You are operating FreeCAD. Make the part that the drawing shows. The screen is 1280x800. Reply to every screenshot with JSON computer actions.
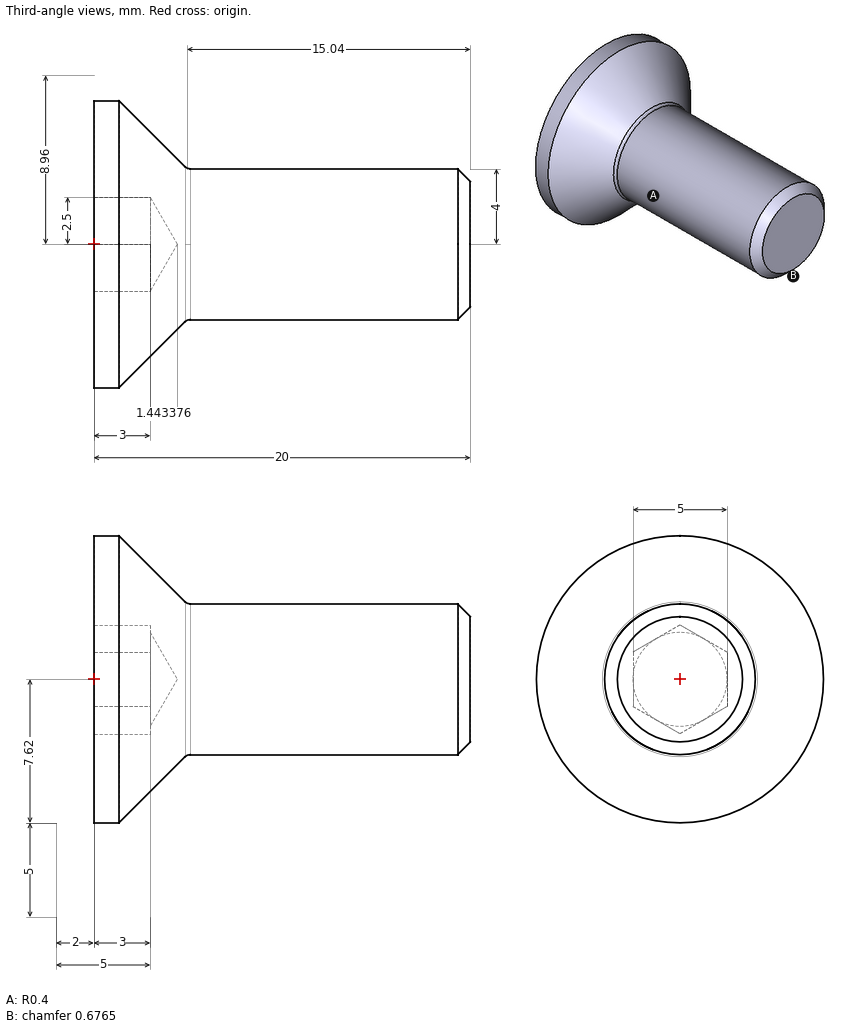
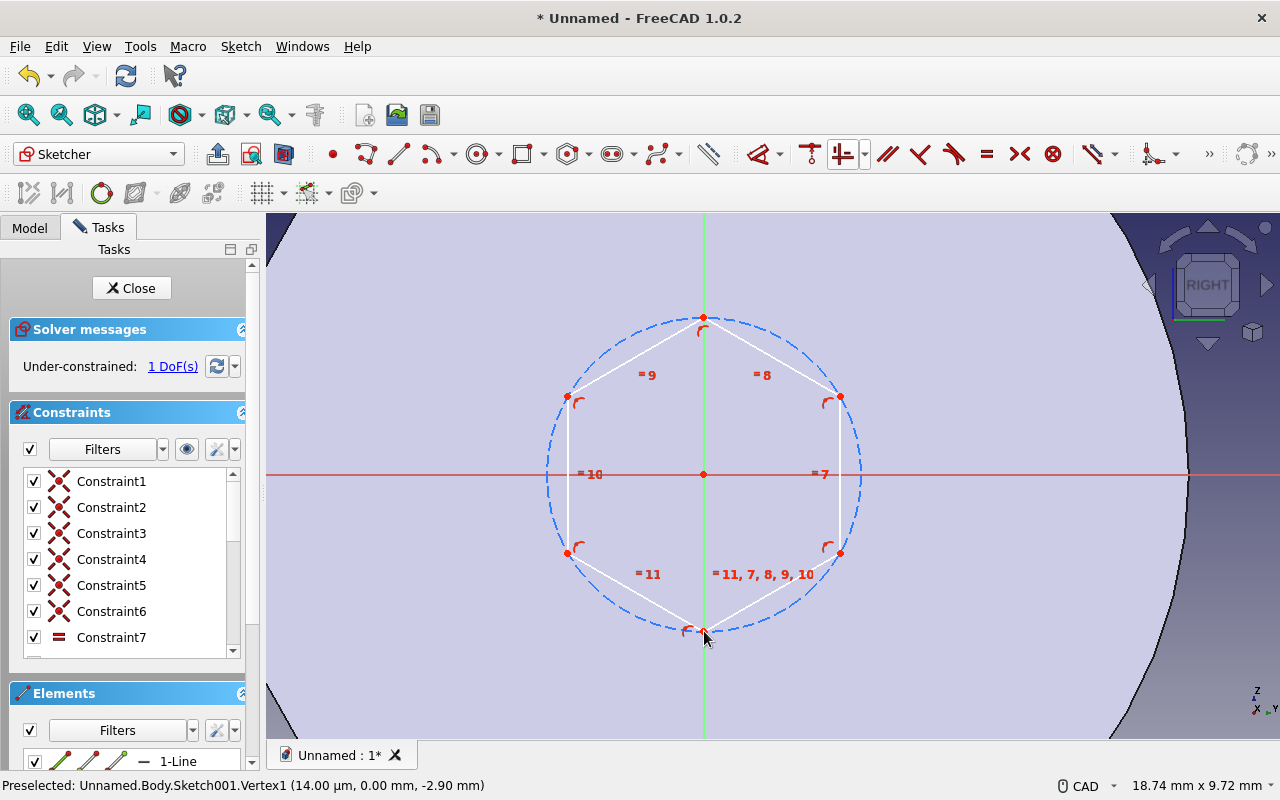
{"action": "left_click", "coordinate": [758, 154]}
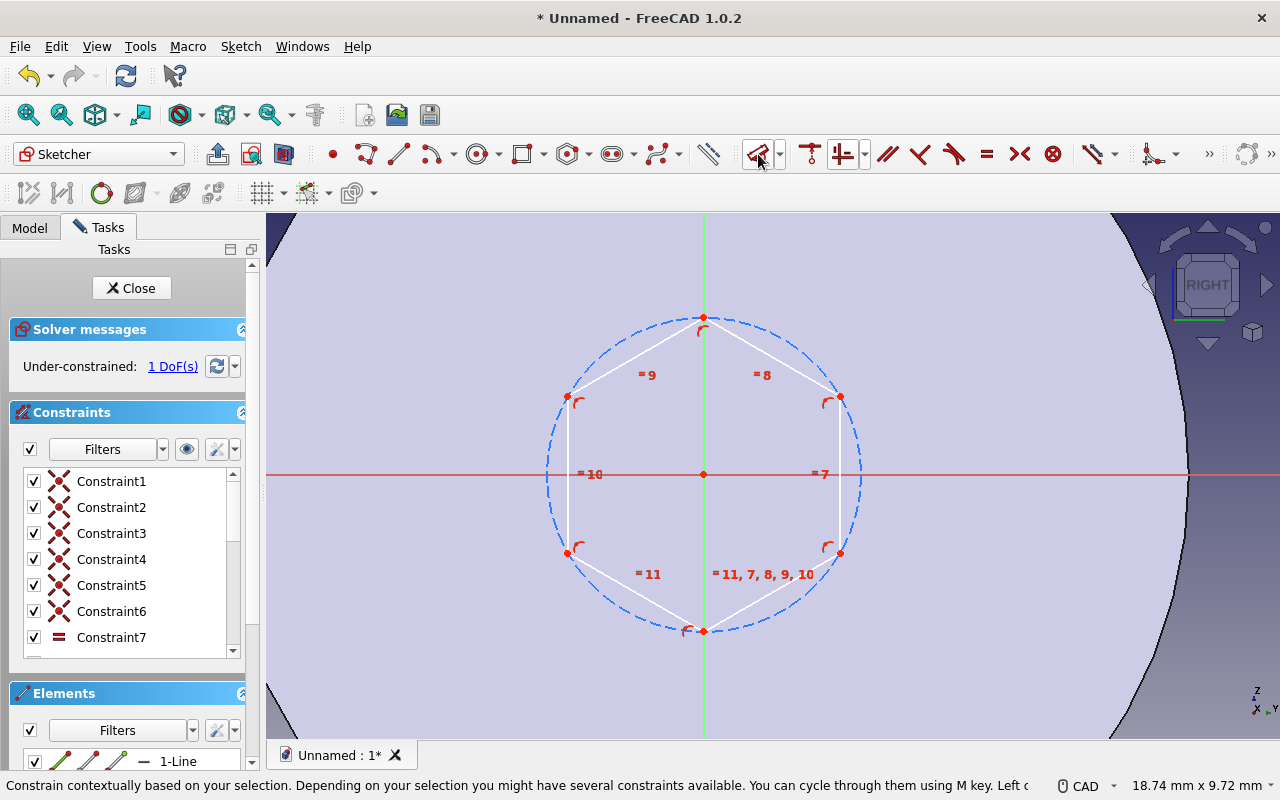
{"action": "left_click", "coordinate": [568, 396]}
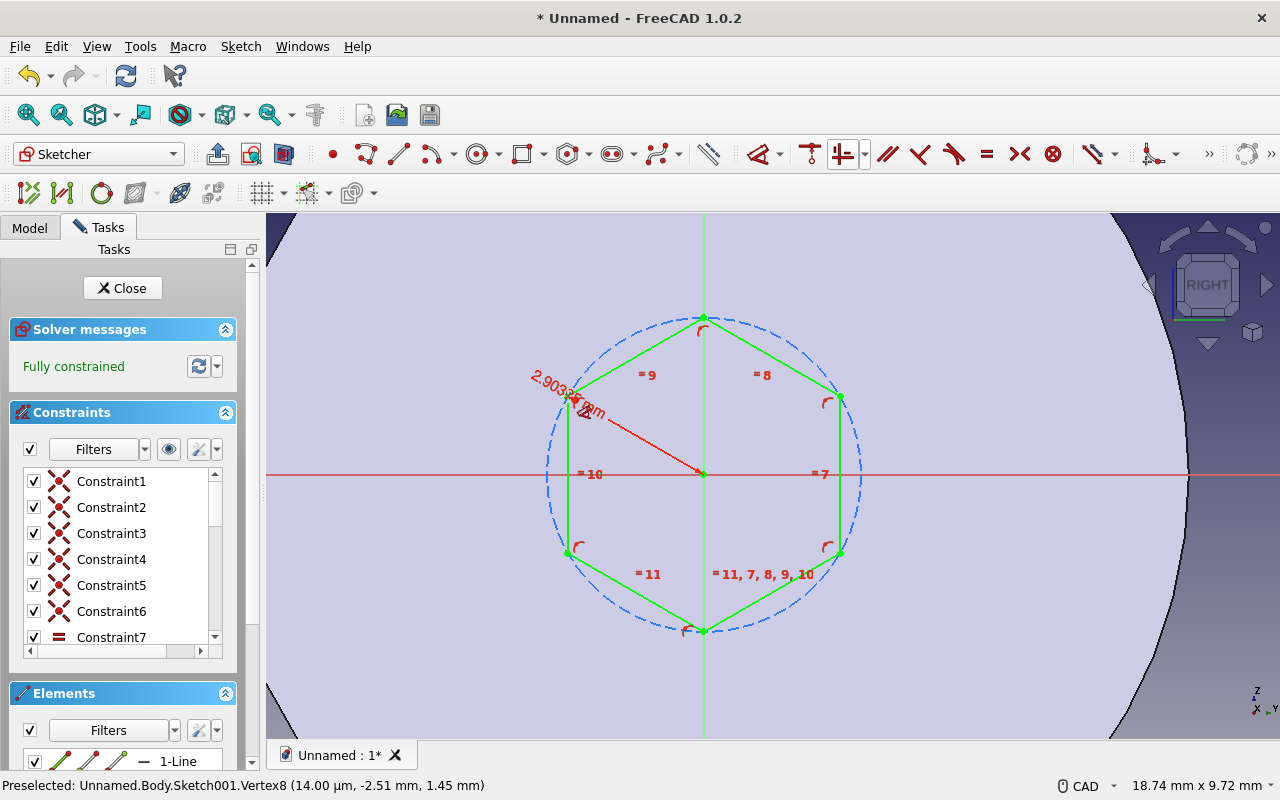
{"action": "left_click", "coordinate": [840, 553]}
{"action": "left_click", "coordinate": [641, 314]}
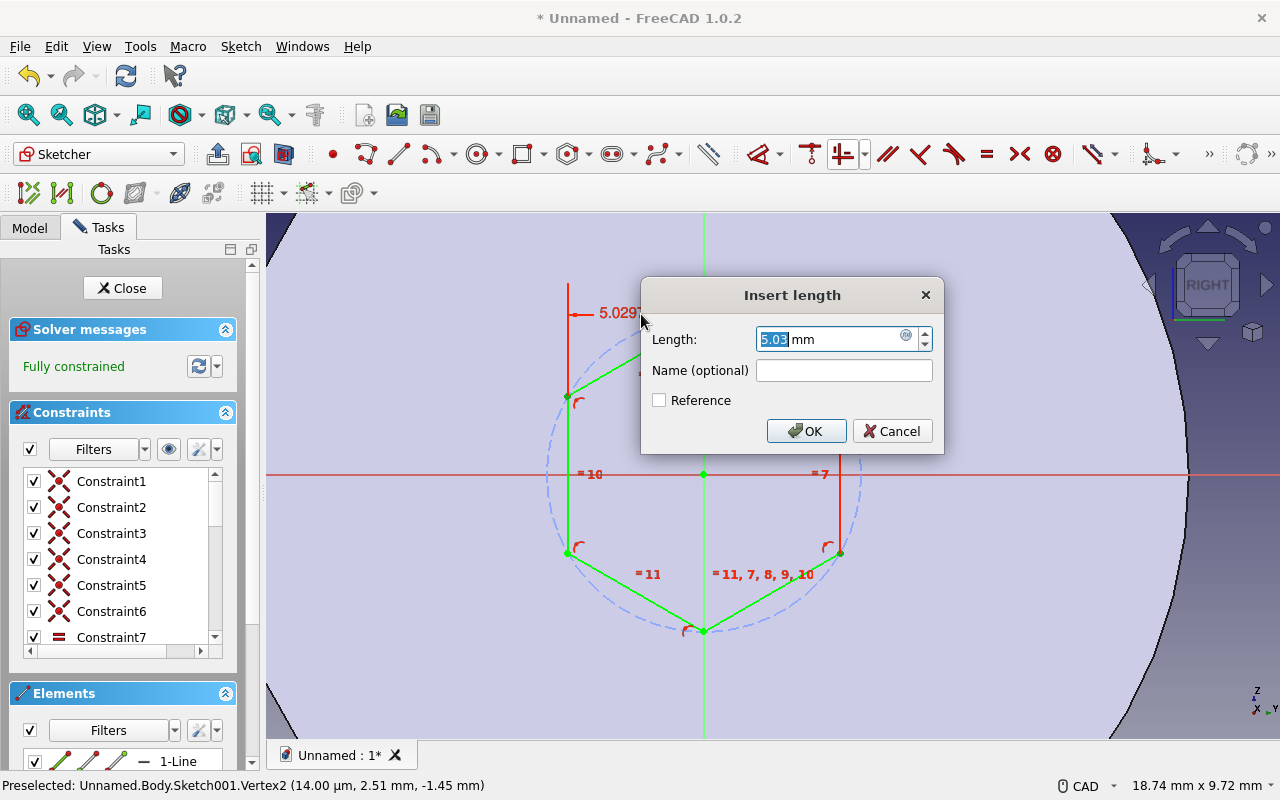
{"action": "type", "text": "5"}
{"action": "key", "text": "Return"}
{"action": "key", "text": "Escape"}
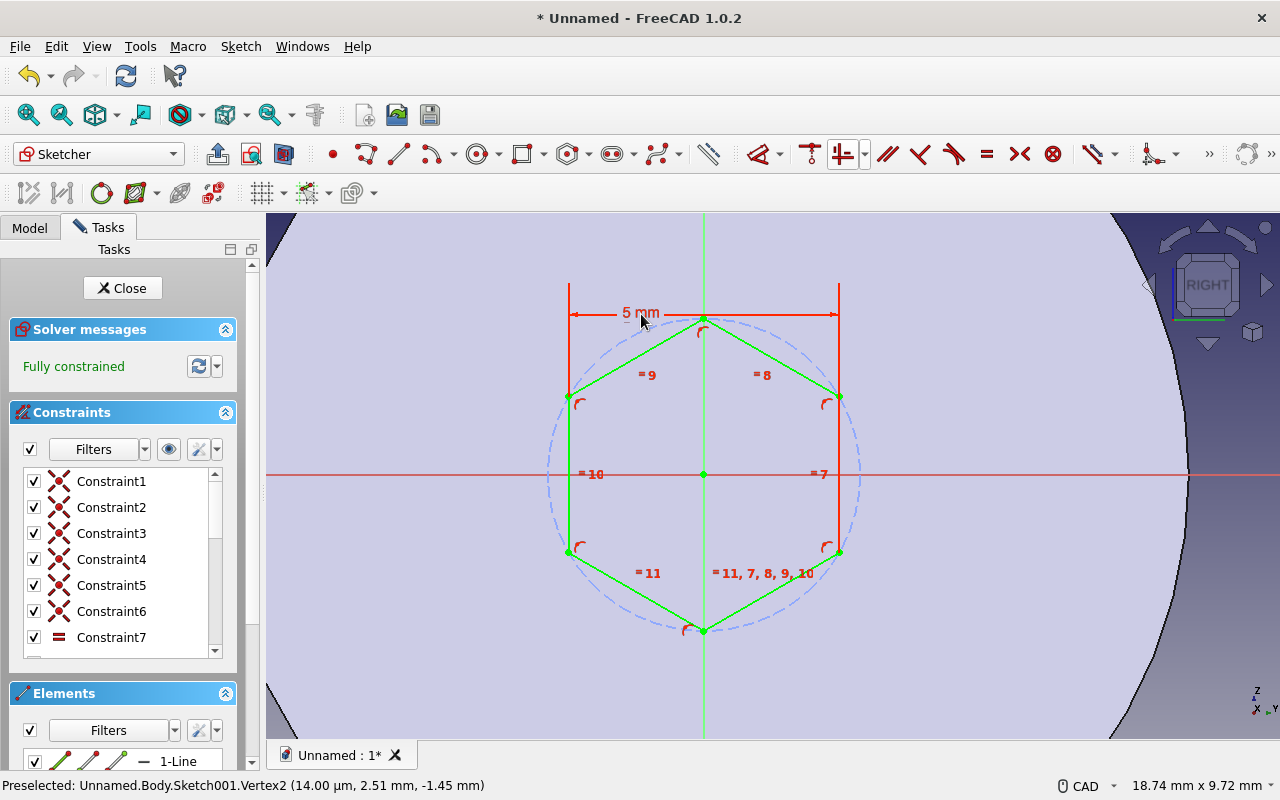
{"action": "left_click", "coordinate": [123, 288]}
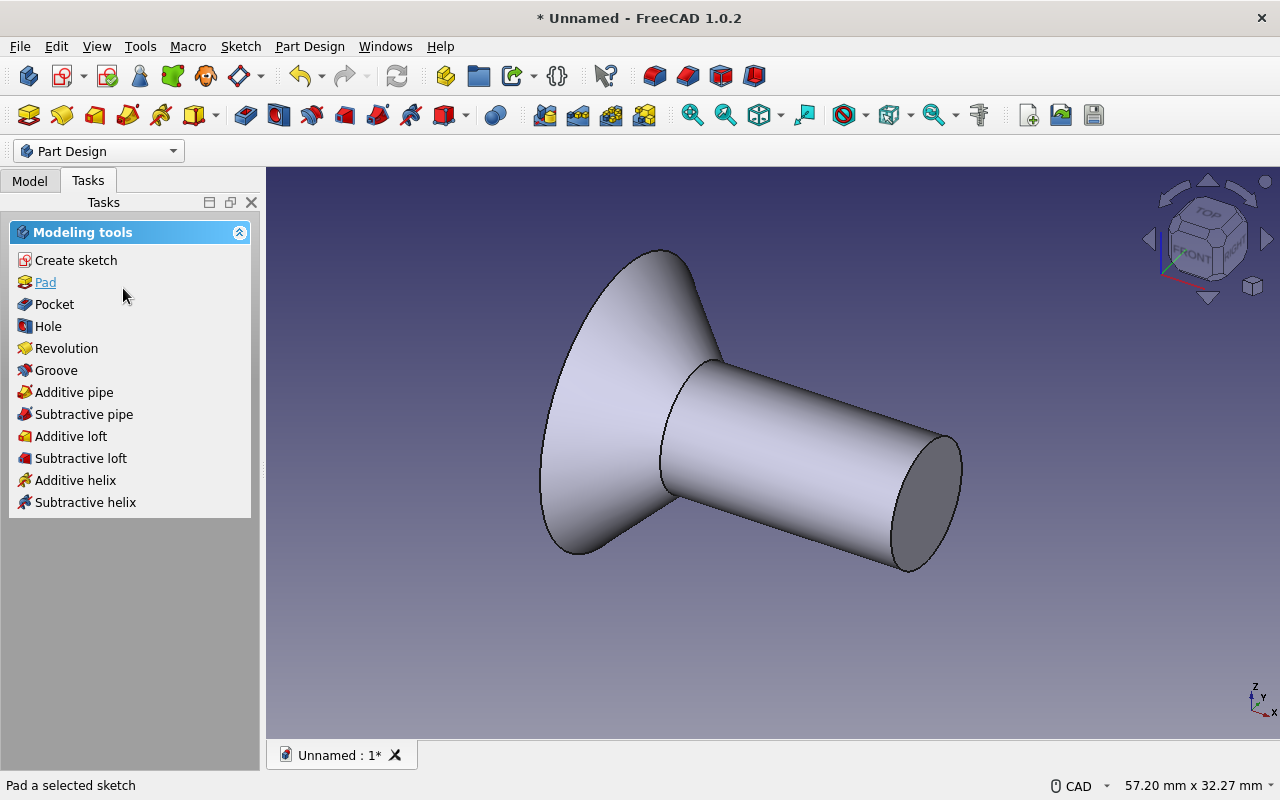
{"action": "left_click", "coordinate": [246, 116]}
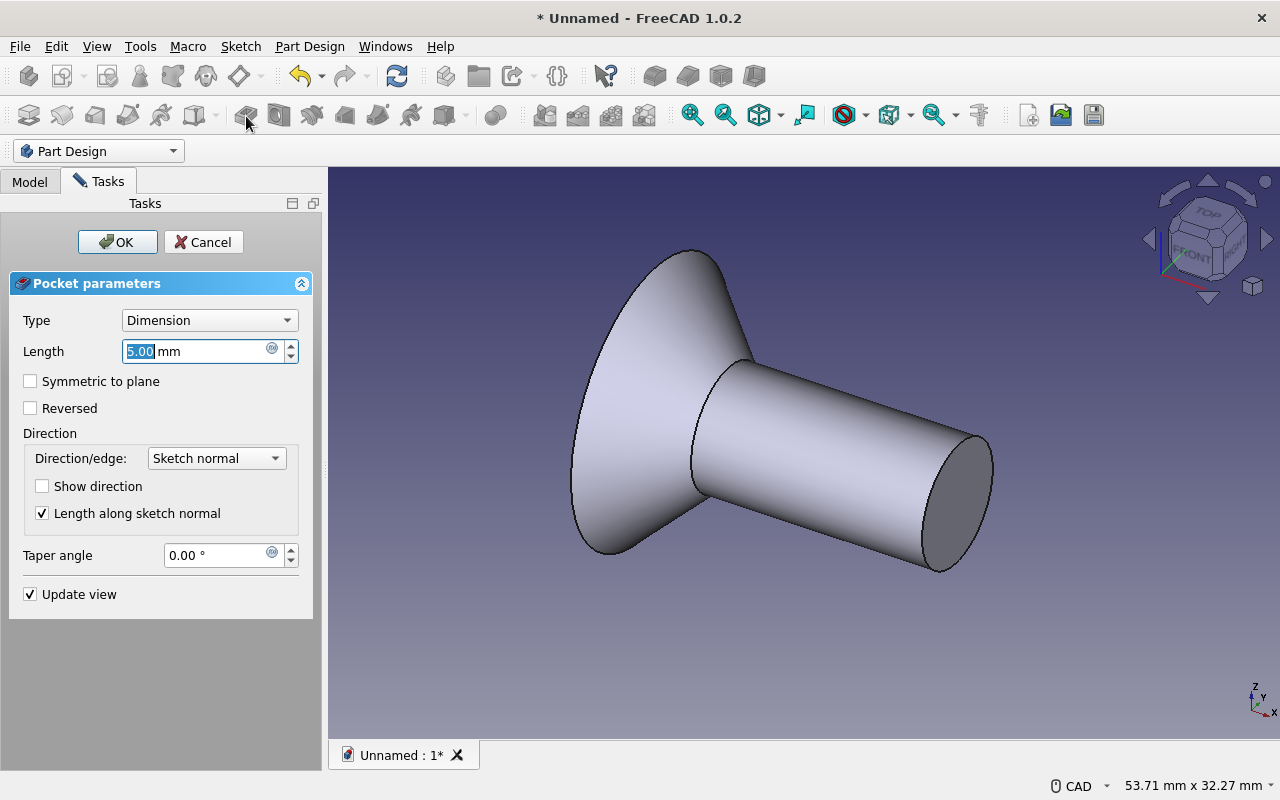
{"action": "type", "text": "3"}
{"action": "key", "text": "Tab"}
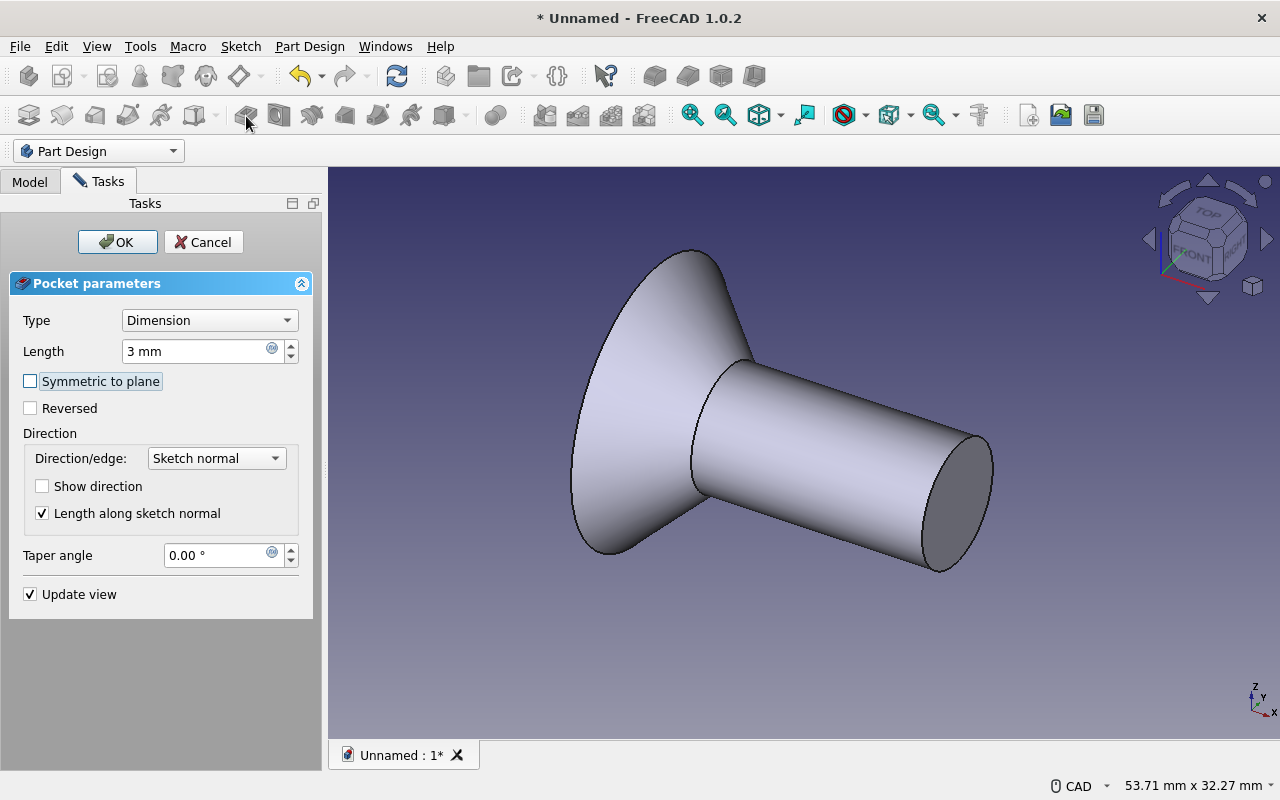
{"action": "left_click", "coordinate": [31, 408]}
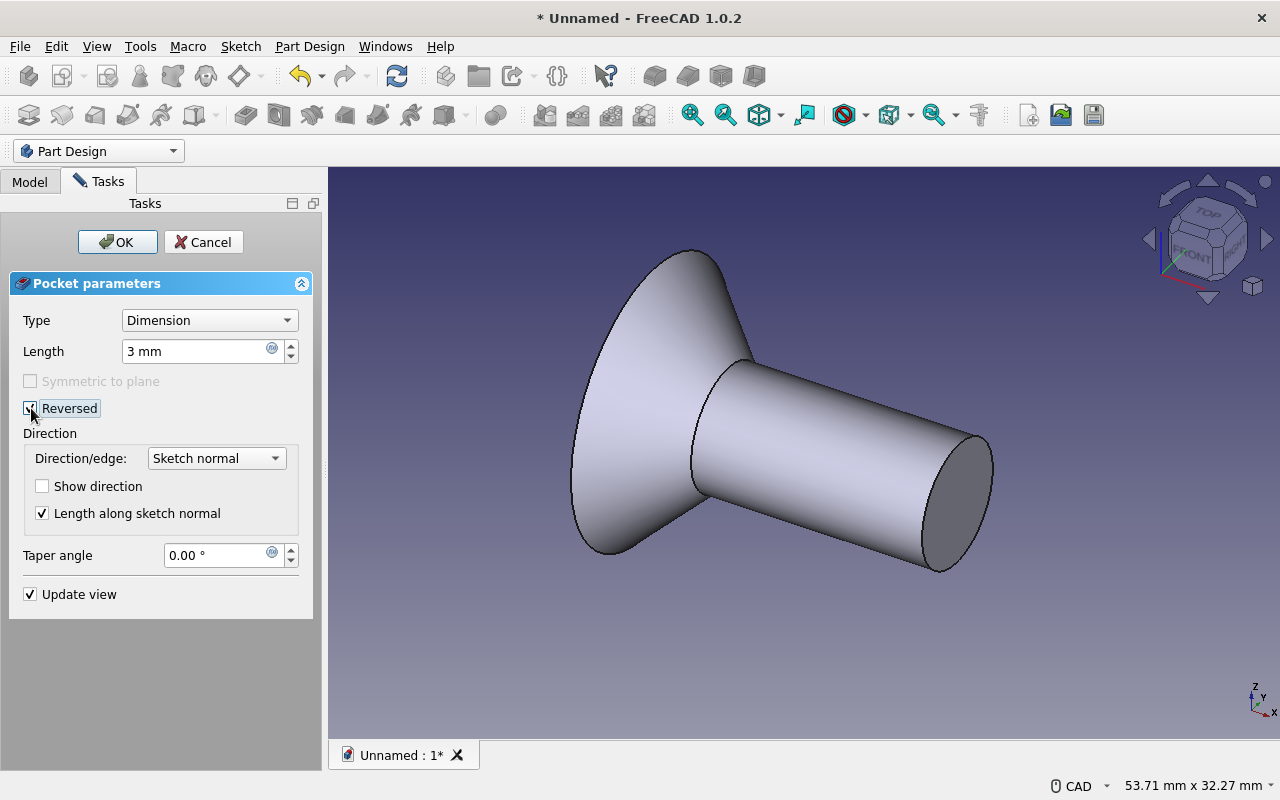
{"action": "left_click", "coordinate": [118, 242]}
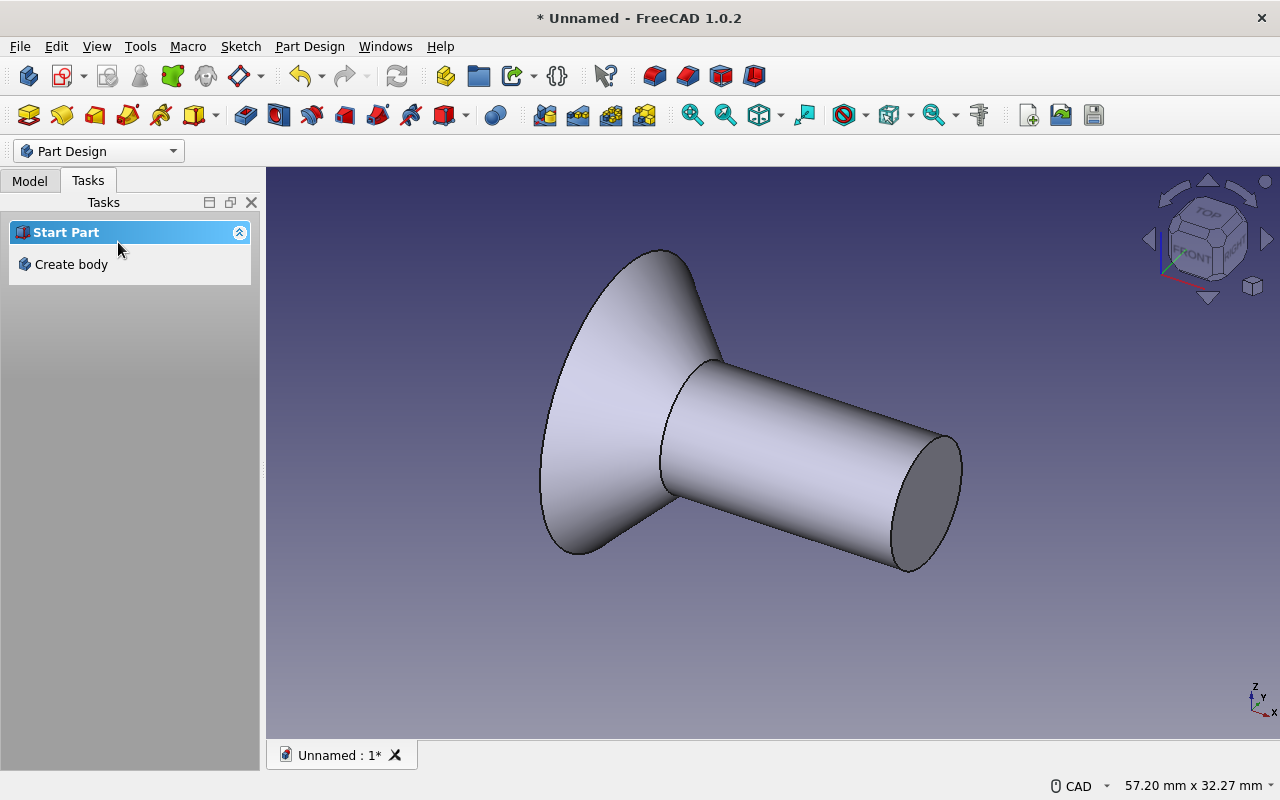
{"action": "left_click", "coordinate": [62, 76]}